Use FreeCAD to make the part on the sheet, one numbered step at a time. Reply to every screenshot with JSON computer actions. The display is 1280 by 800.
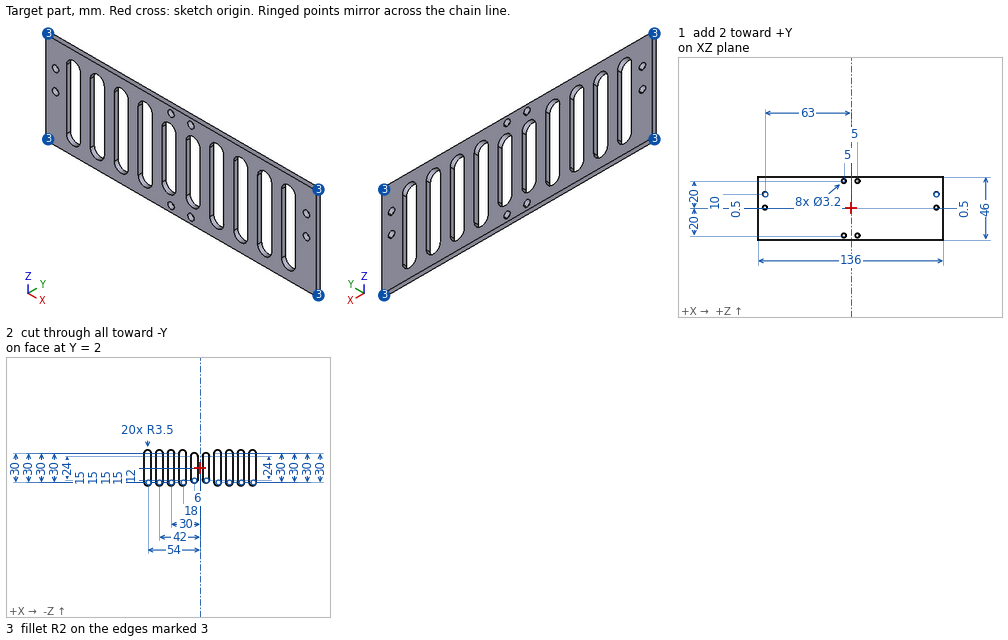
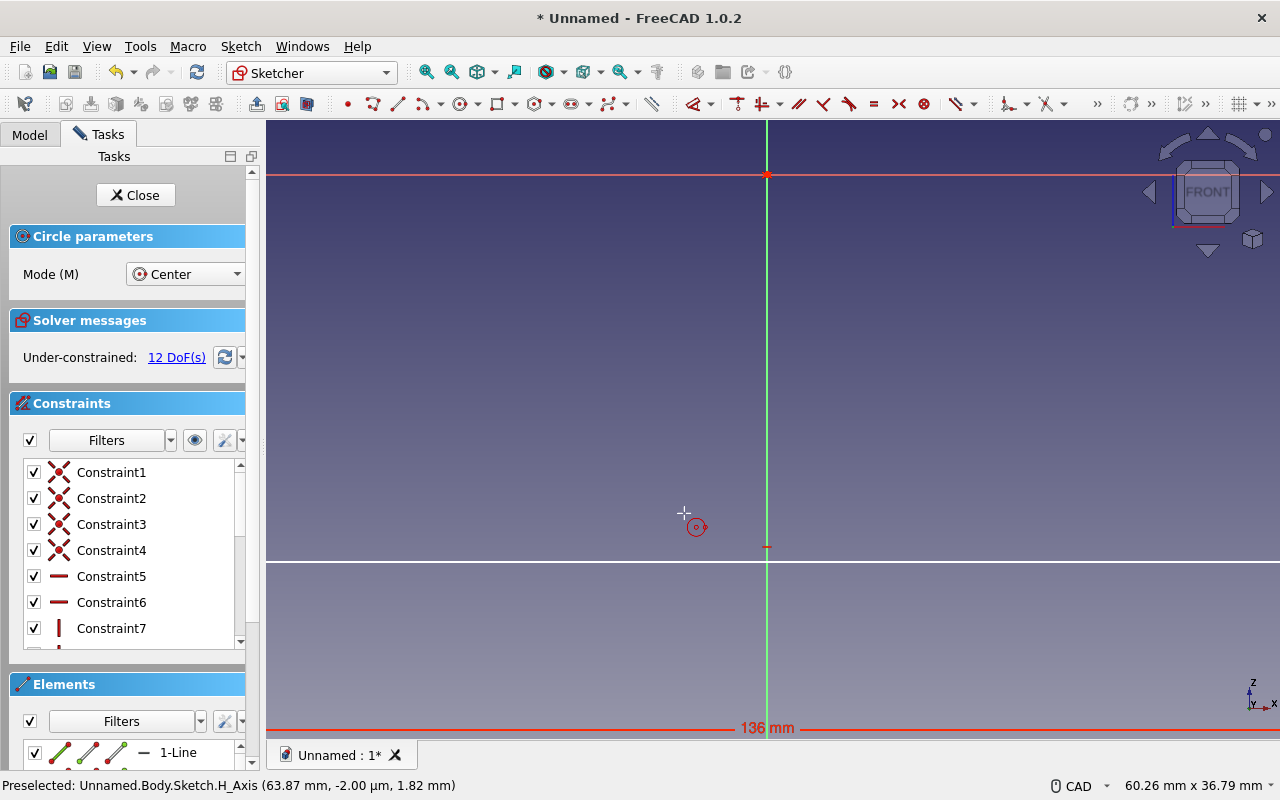
{"action": "scroll", "coordinate": [684, 513], "scroll_direction": "down", "scroll_amount": 7}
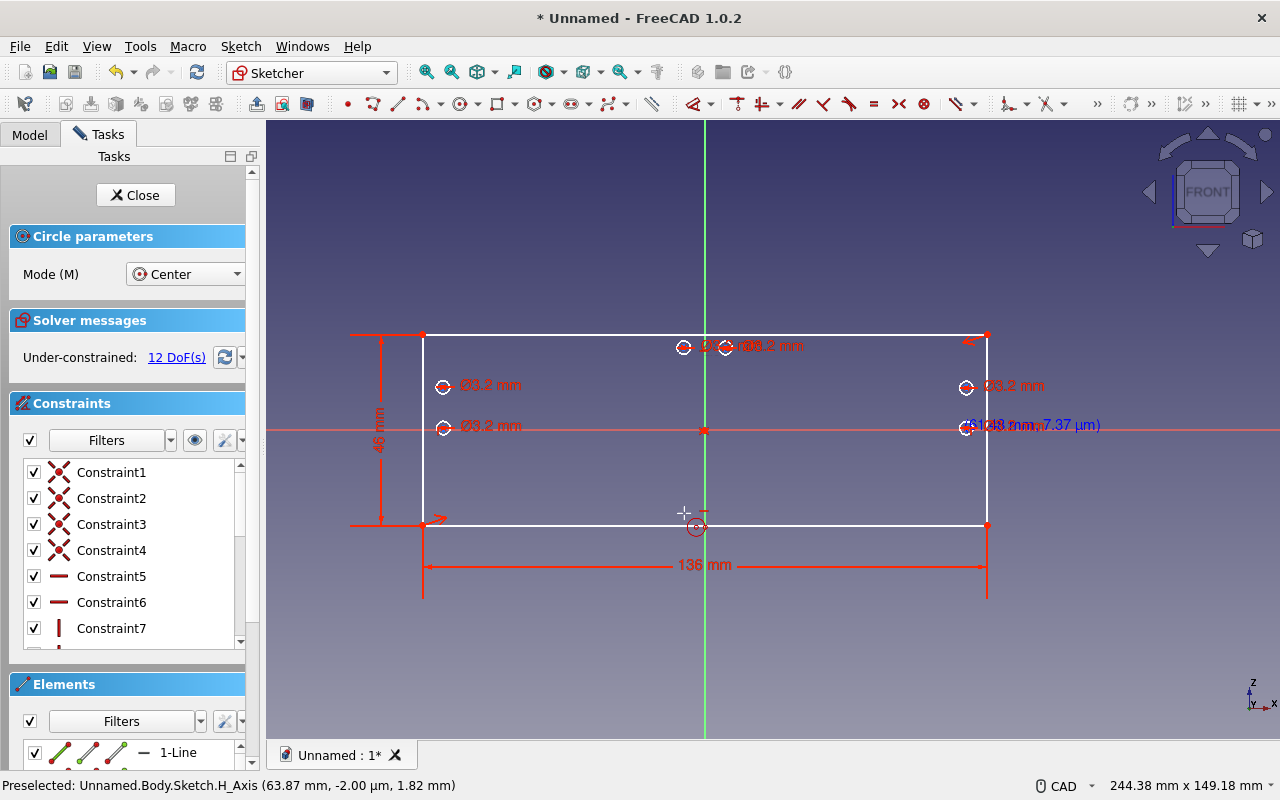
{"action": "scroll", "coordinate": [684, 513], "scroll_direction": "up", "scroll_amount": 2}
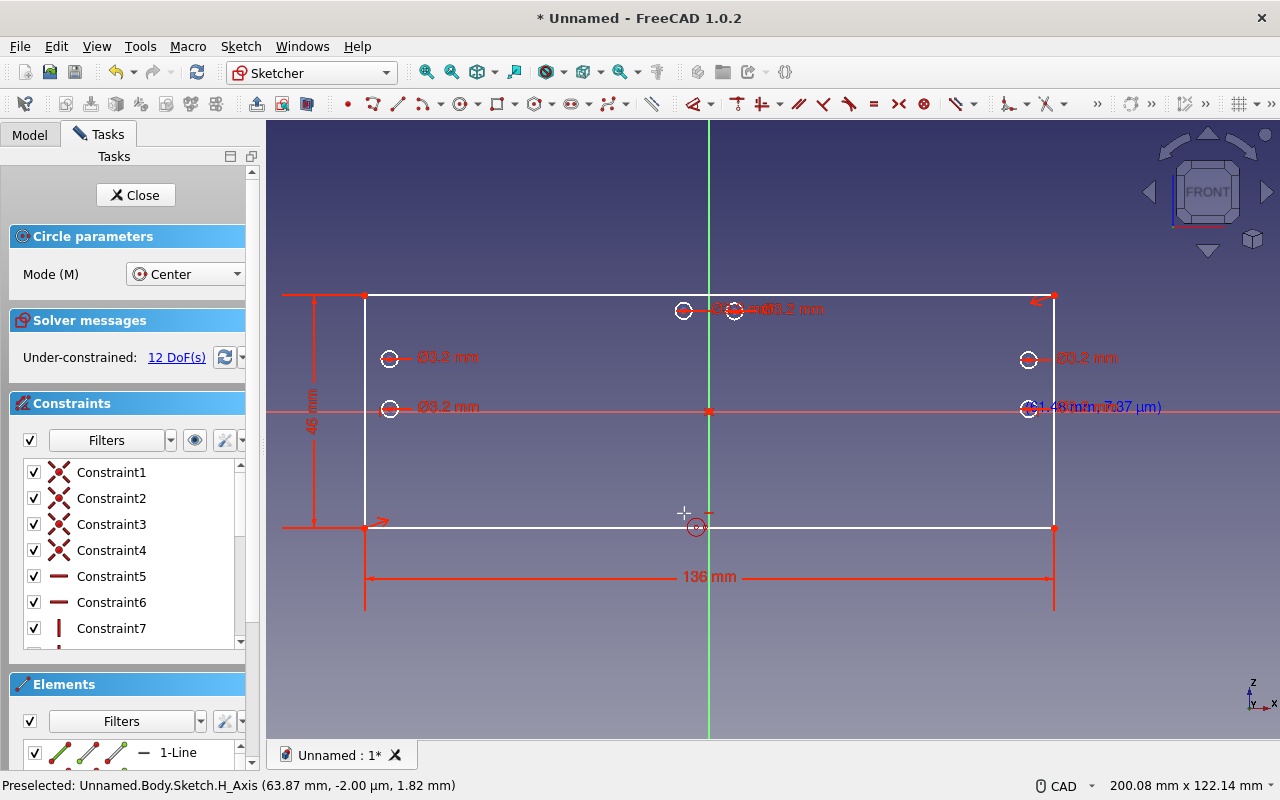
{"action": "left_click", "coordinate": [684, 513]}
{"action": "mouse_move", "coordinate": [691, 506]}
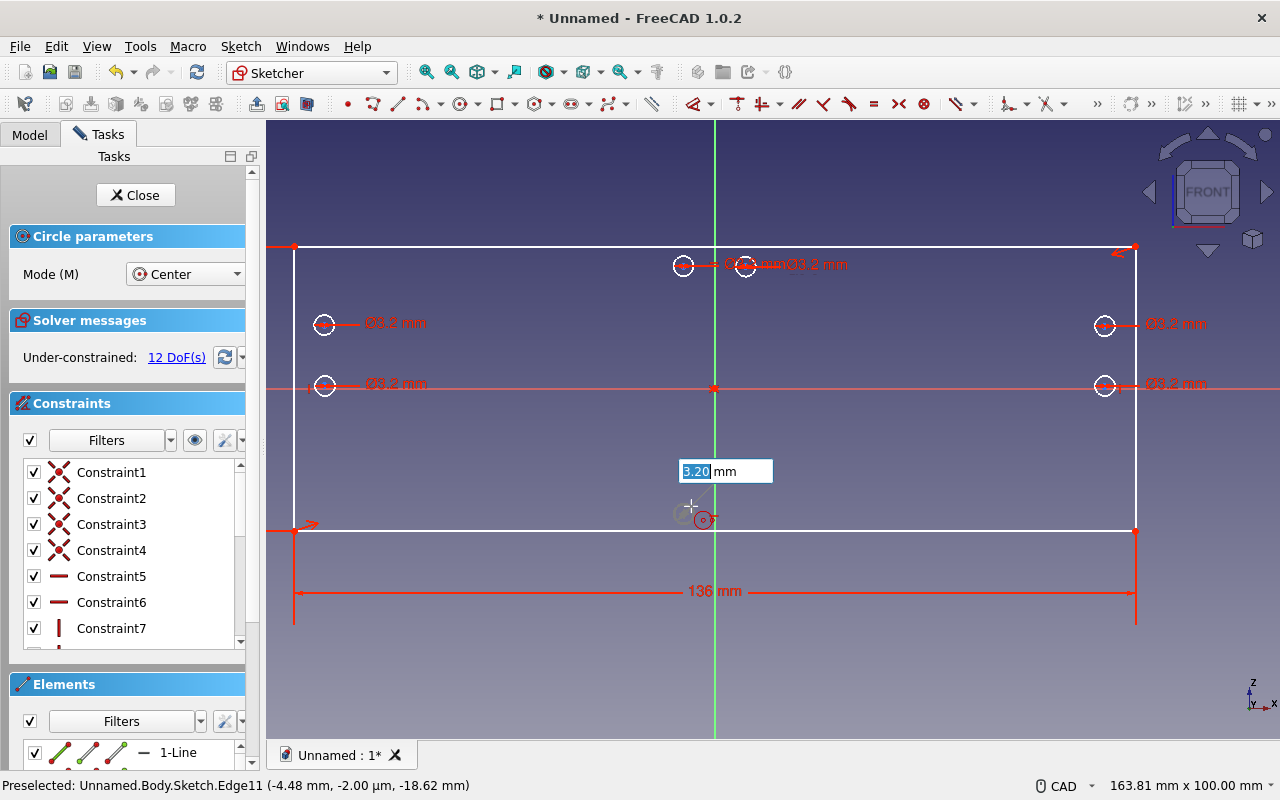
{"action": "type", "text": "3.2"}
{"action": "key", "text": "Return"}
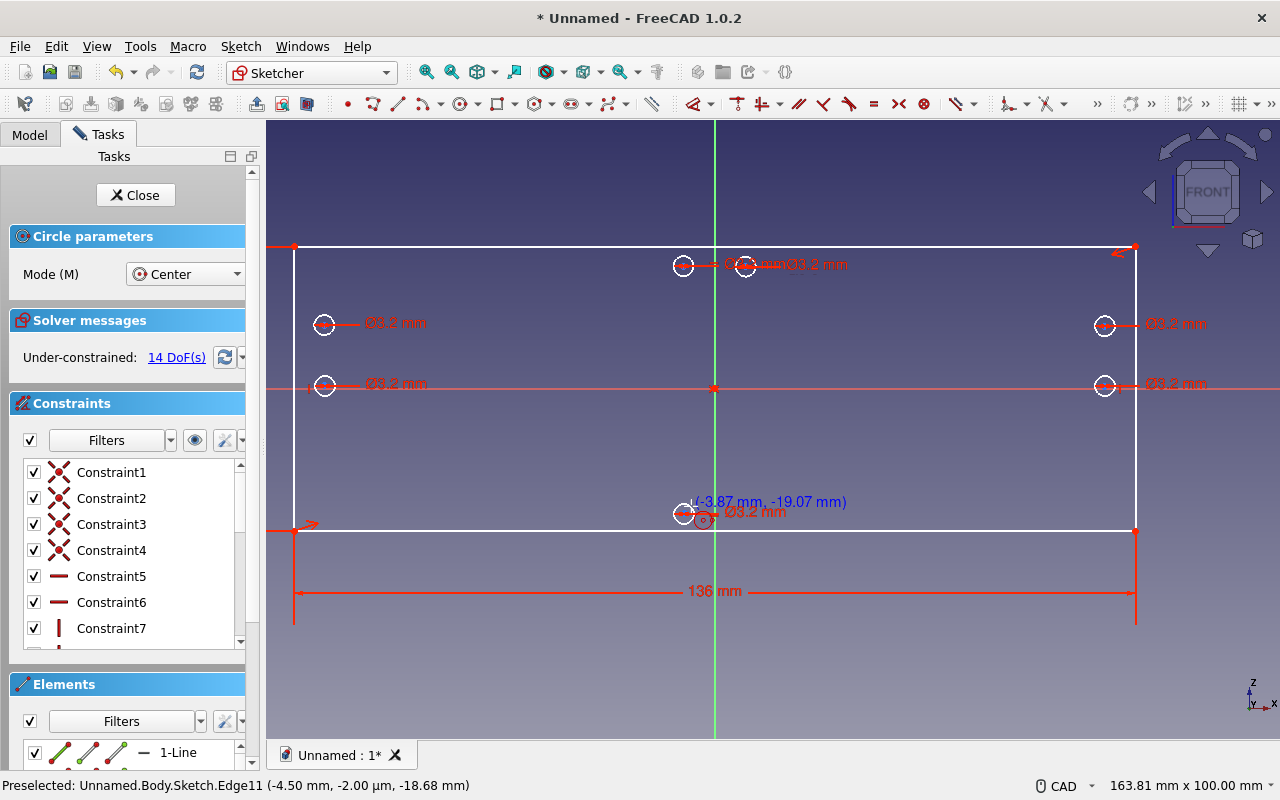
{"action": "scroll", "coordinate": [746, 513], "scroll_direction": "up", "scroll_amount": 5}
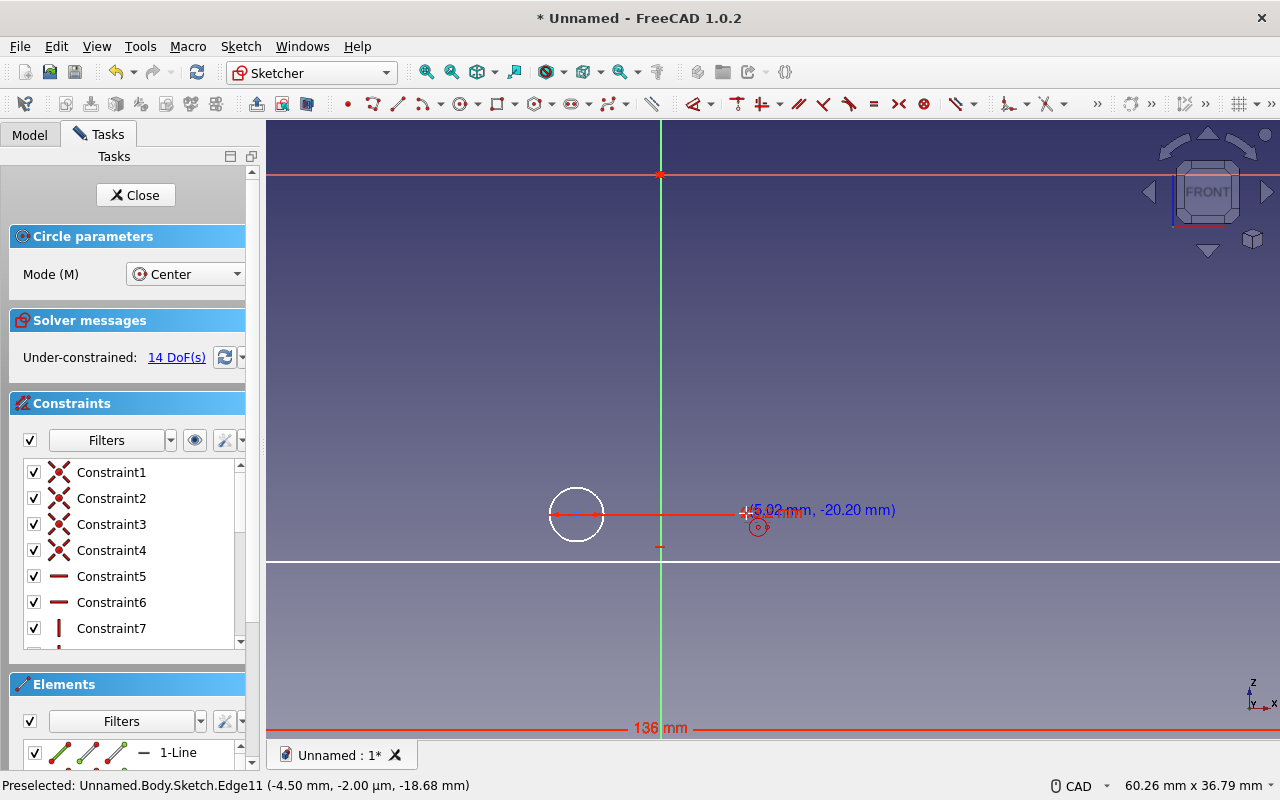
{"action": "scroll", "coordinate": [719, 513], "scroll_direction": "down", "scroll_amount": 7}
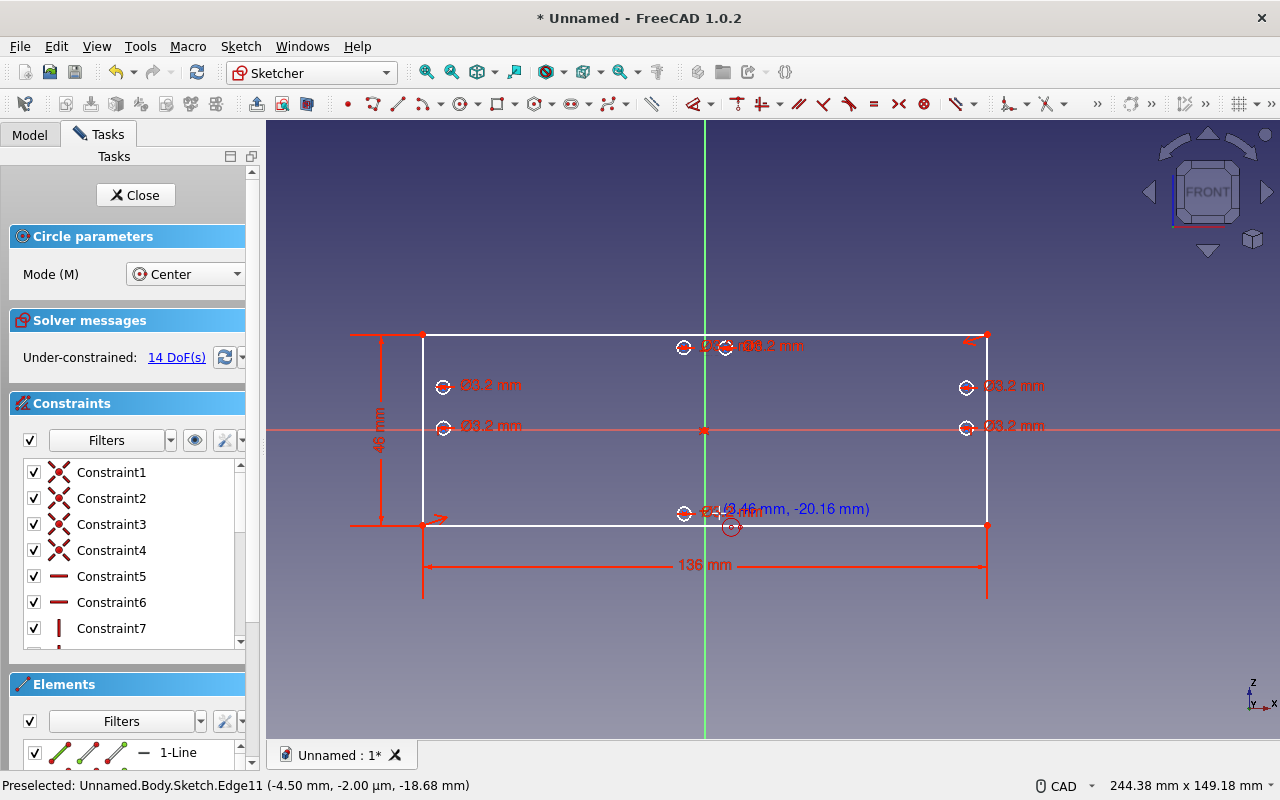
{"action": "scroll", "coordinate": [726, 513], "scroll_direction": "up", "scroll_amount": 2}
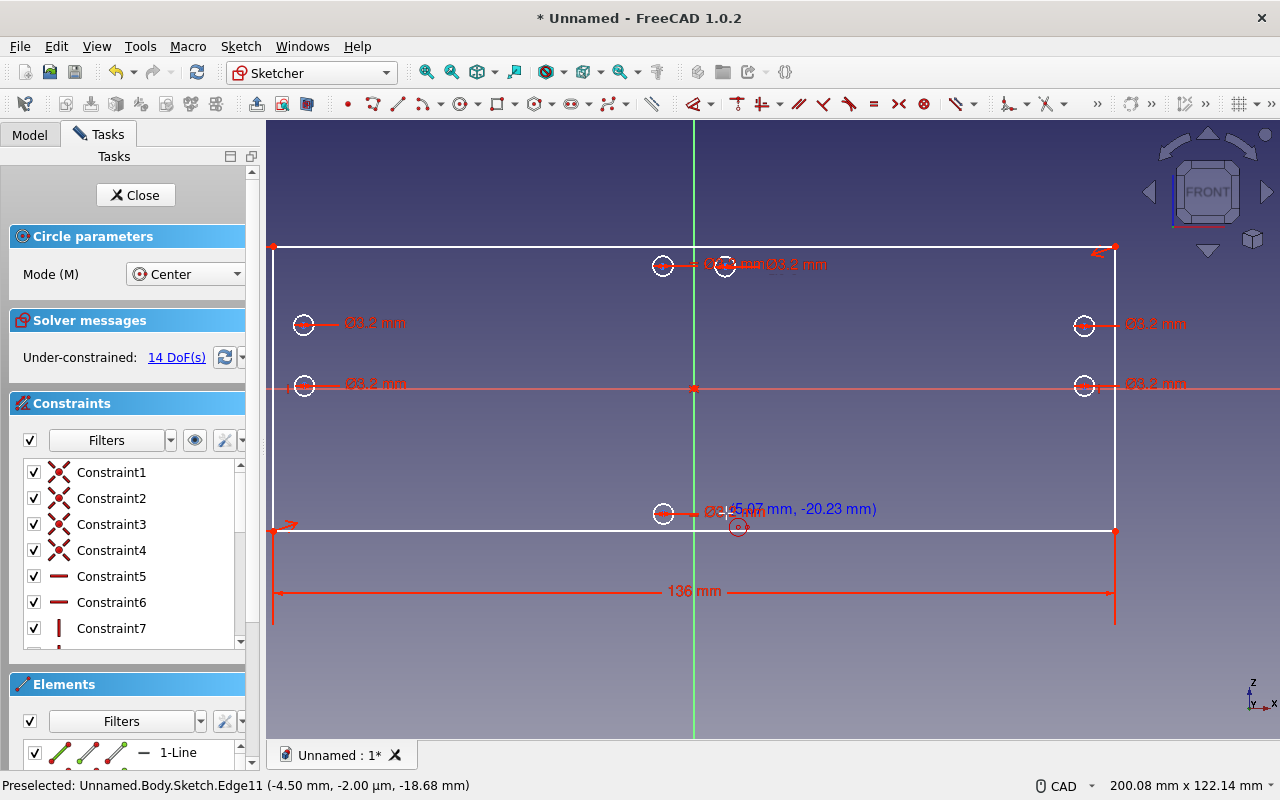
{"action": "left_click", "coordinate": [725, 513]}
{"action": "mouse_move", "coordinate": [732, 506]}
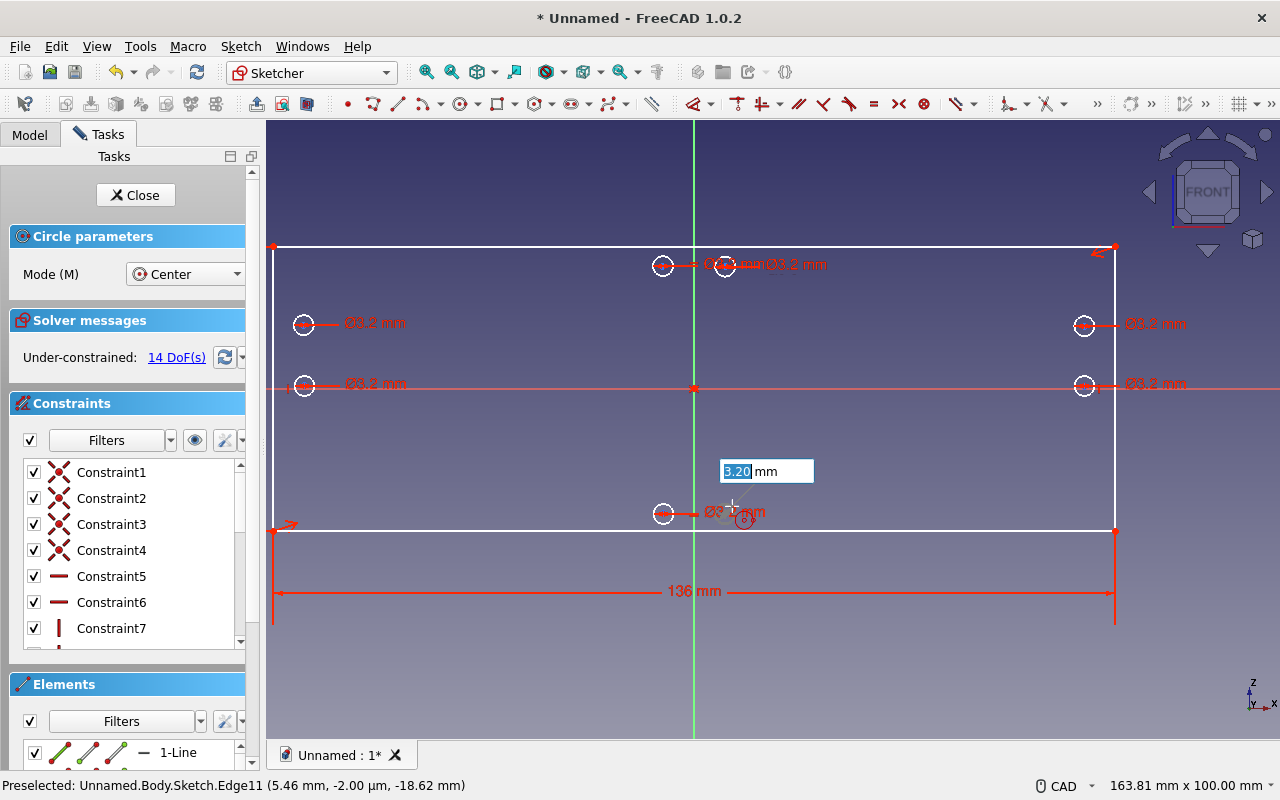
{"action": "type", "text": "3.2"}
{"action": "key", "text": "Return"}
{"action": "key", "text": "Escape"}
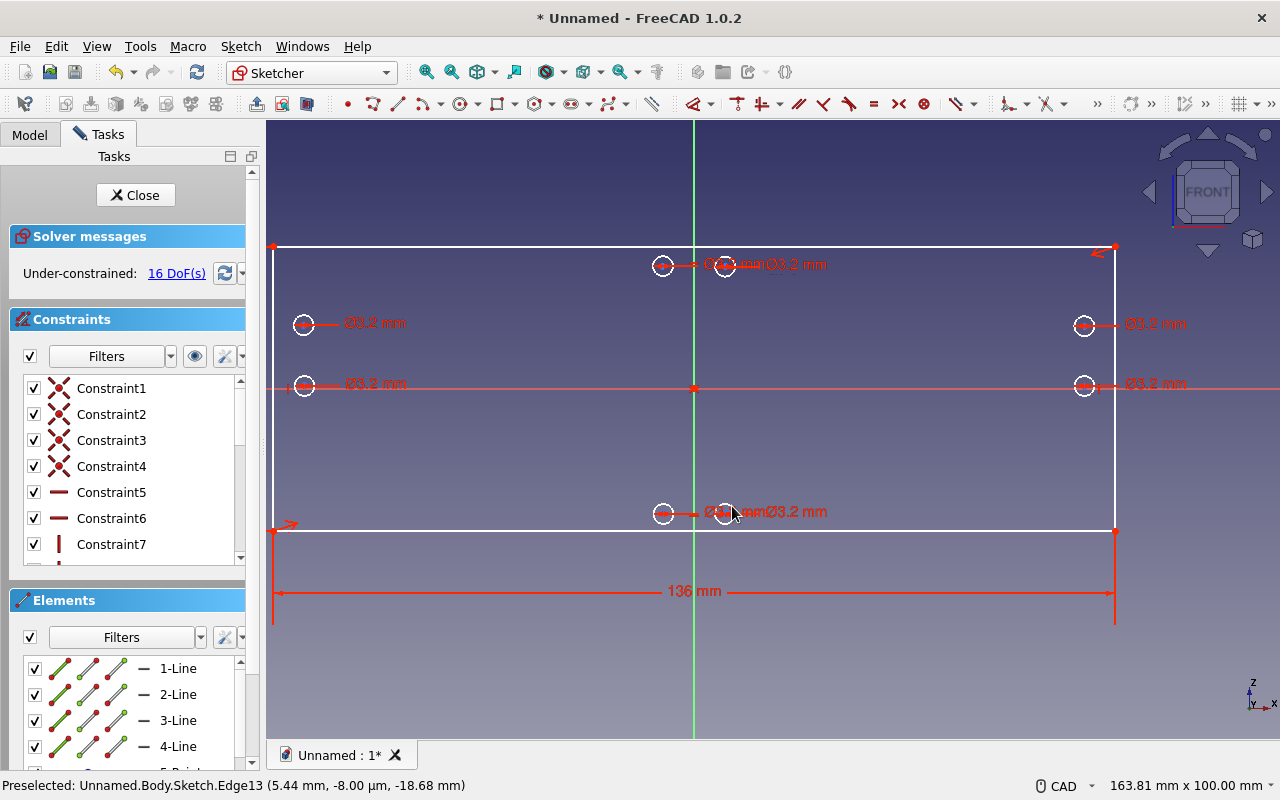
{"action": "left_click", "coordinate": [304, 325]}